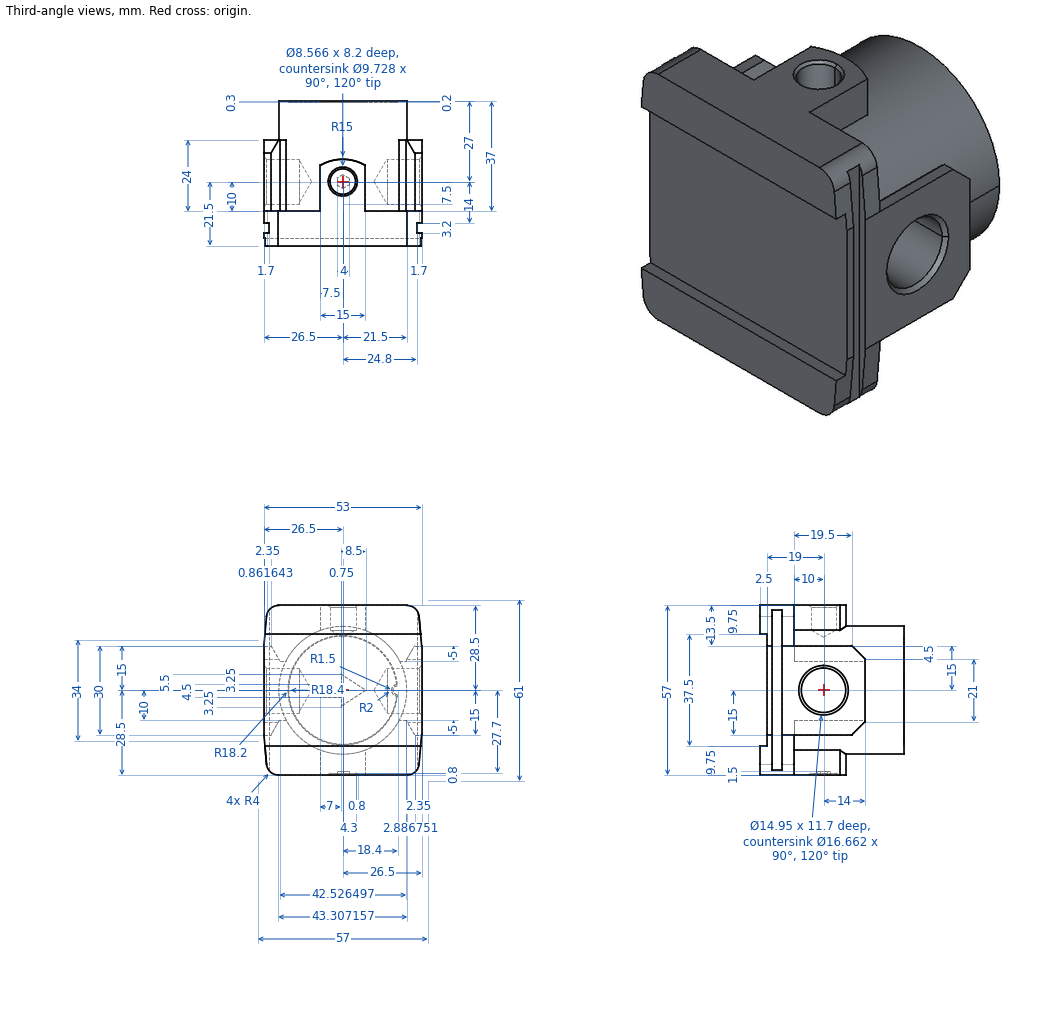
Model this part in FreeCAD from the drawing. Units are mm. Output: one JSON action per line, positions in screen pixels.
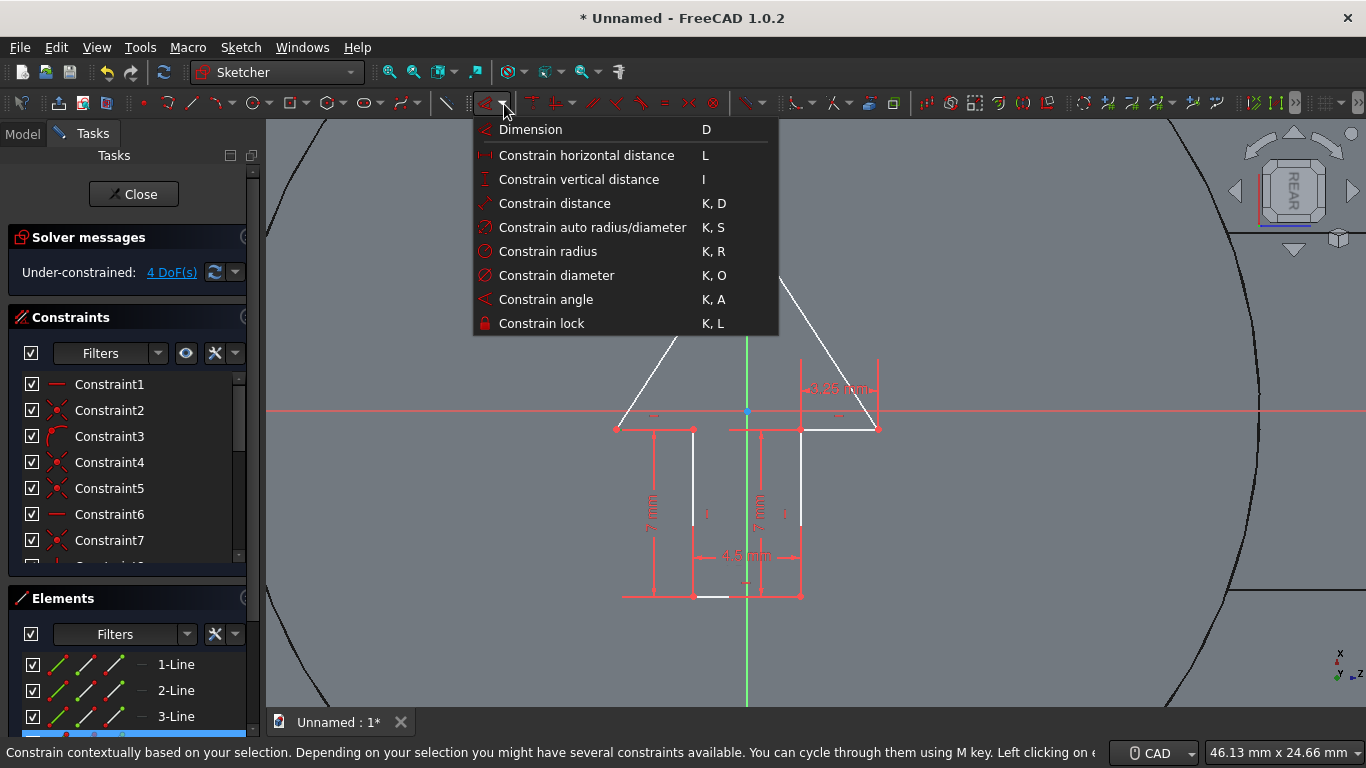
{"action": "left_click", "coordinate": [626, 155]}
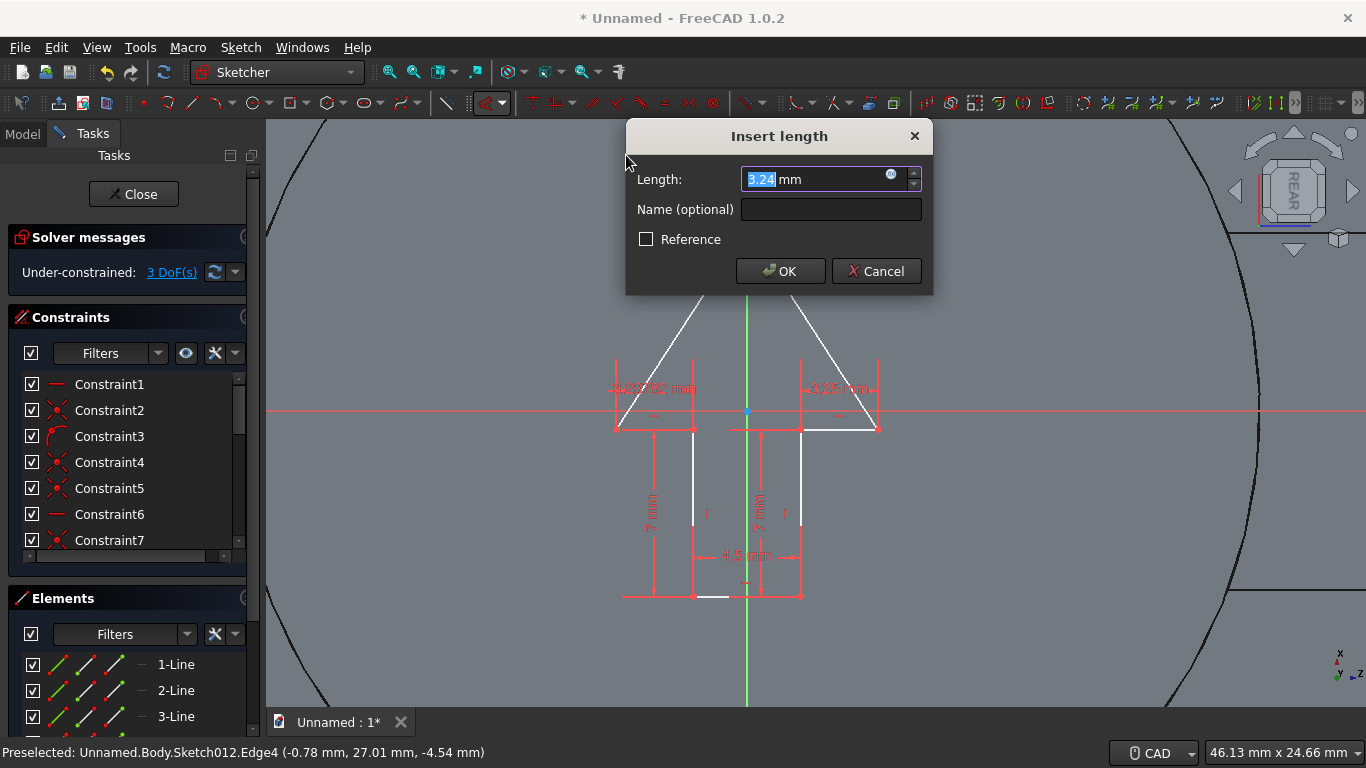
{"action": "type", "text": "3.25"}
{"action": "key", "text": "Return"}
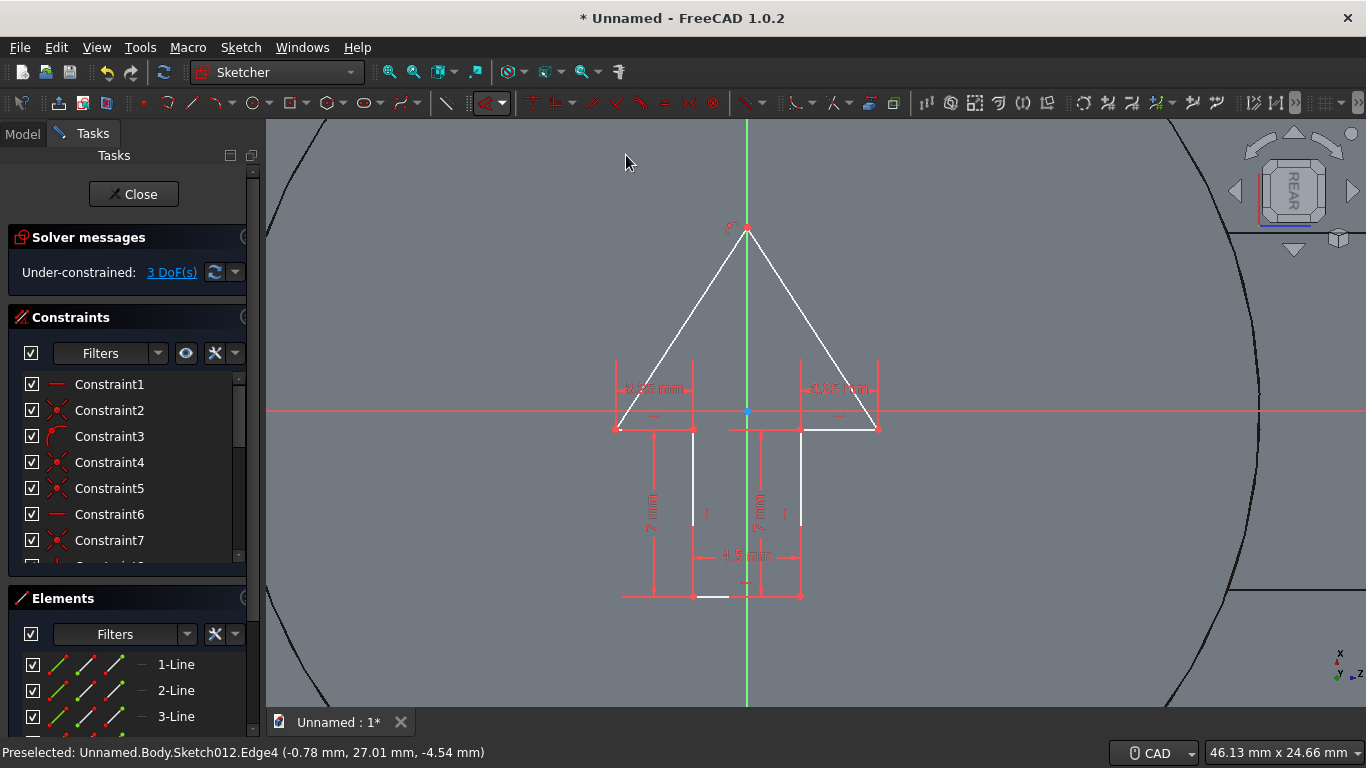
{"action": "left_click", "coordinate": [878, 430]}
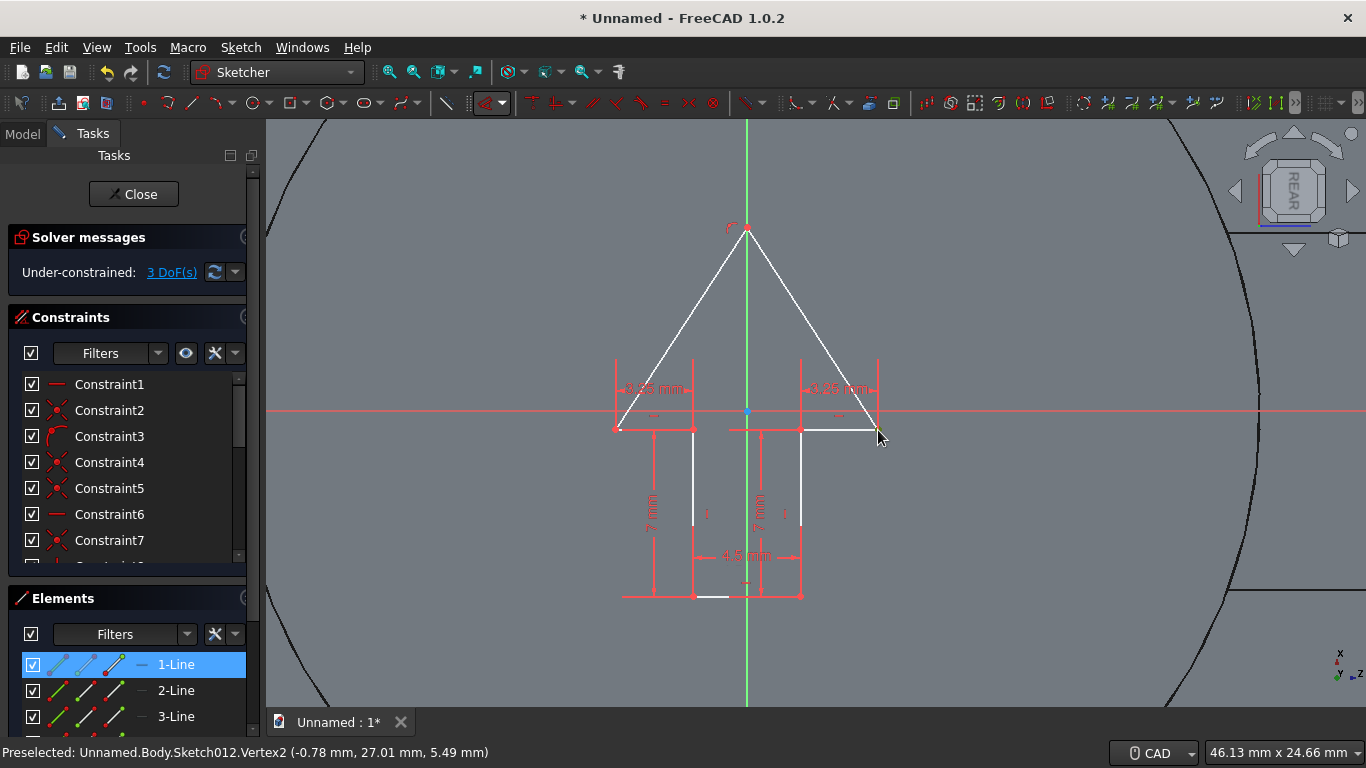
{"action": "key", "text": "l"}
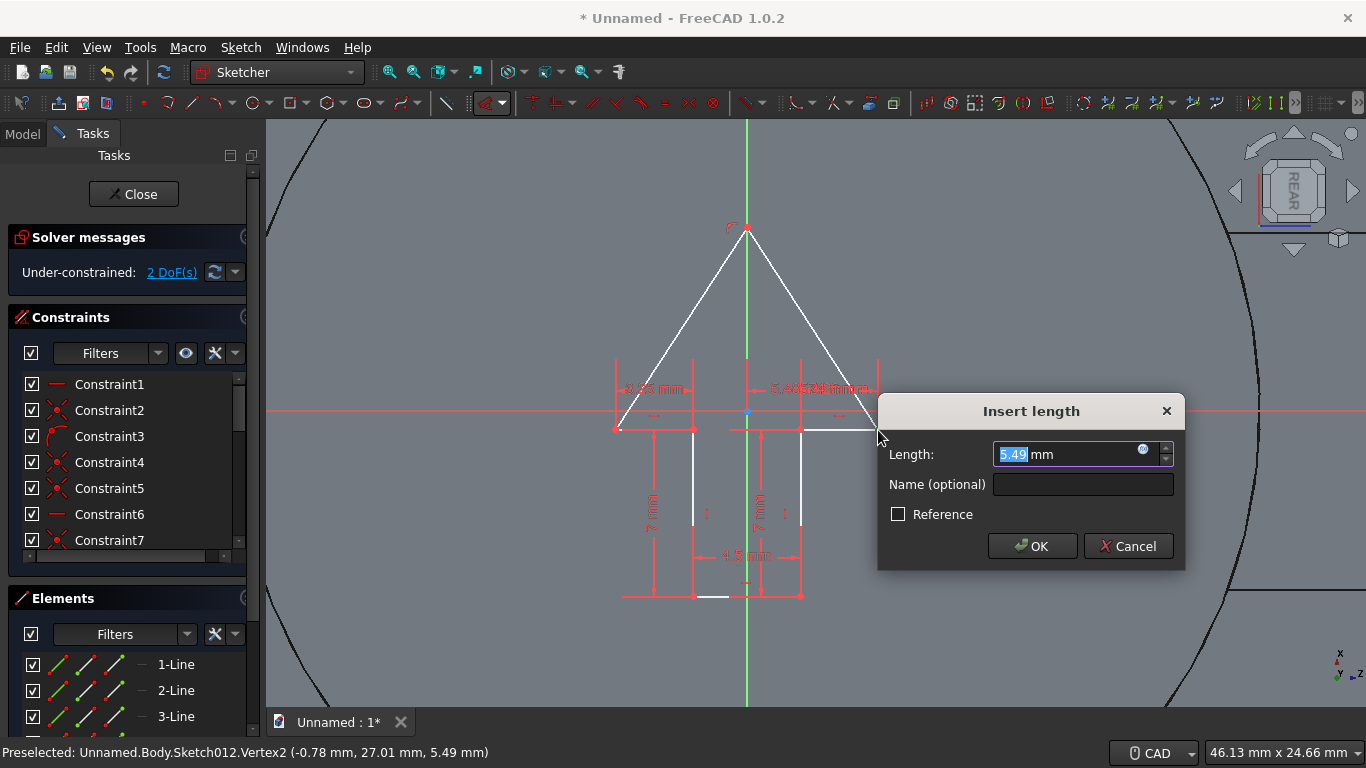
{"action": "type", "text": "5.5"}
{"action": "key", "text": "Return"}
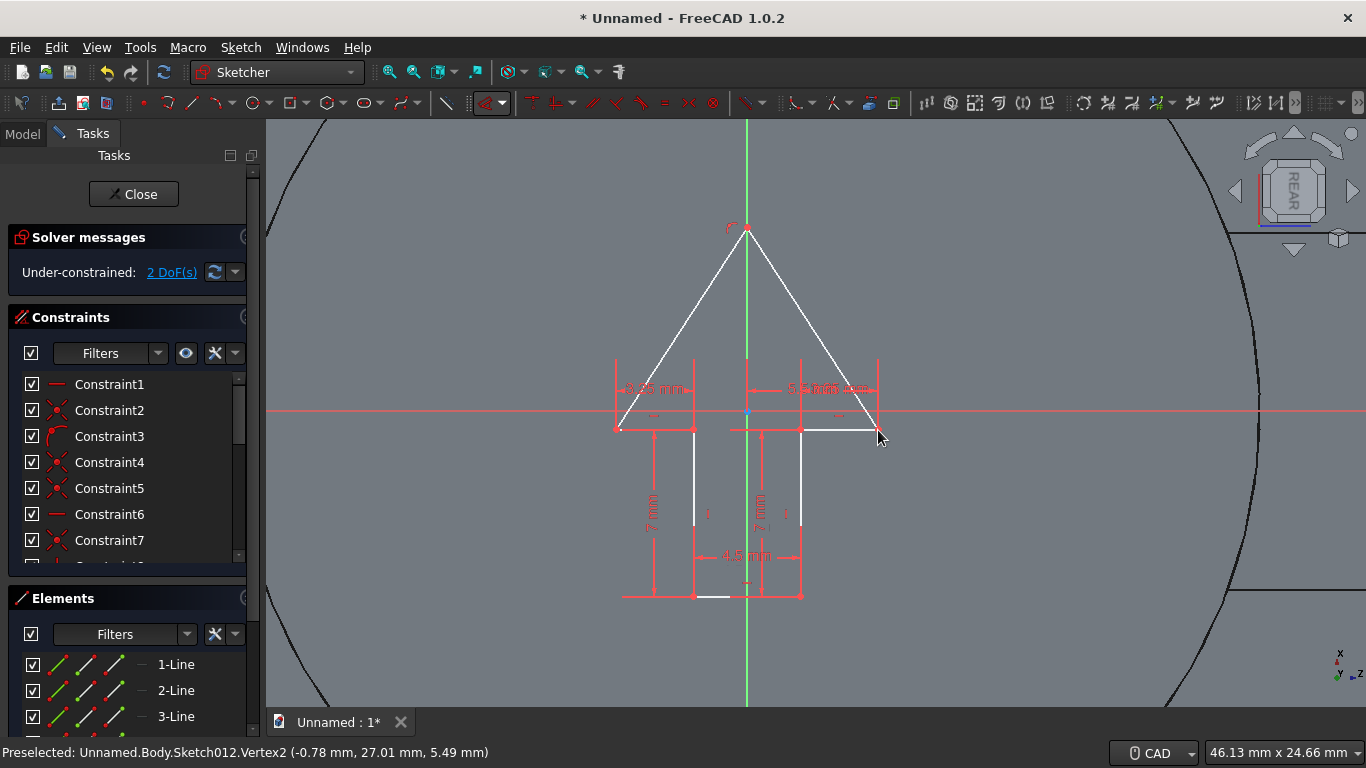
{"action": "left_click", "coordinate": [839, 369]}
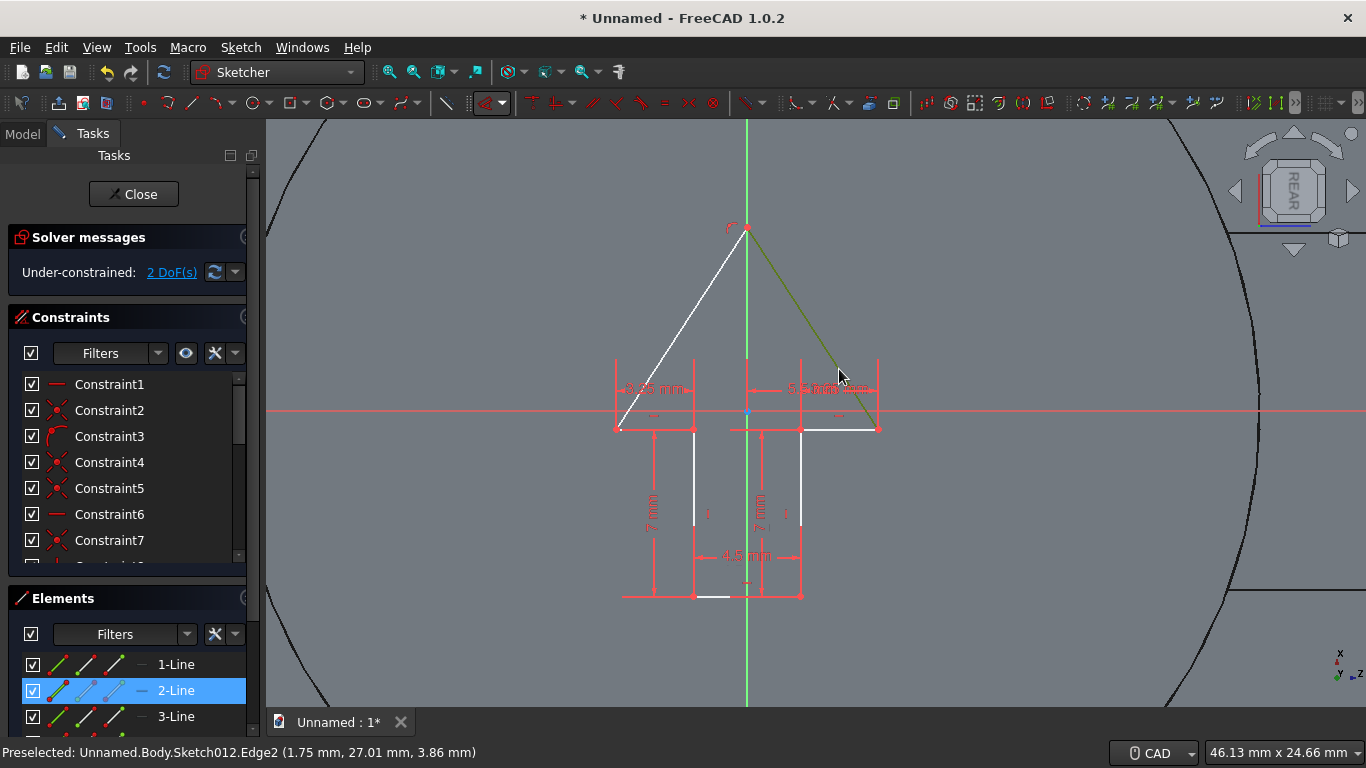
{"action": "key", "text": "i"}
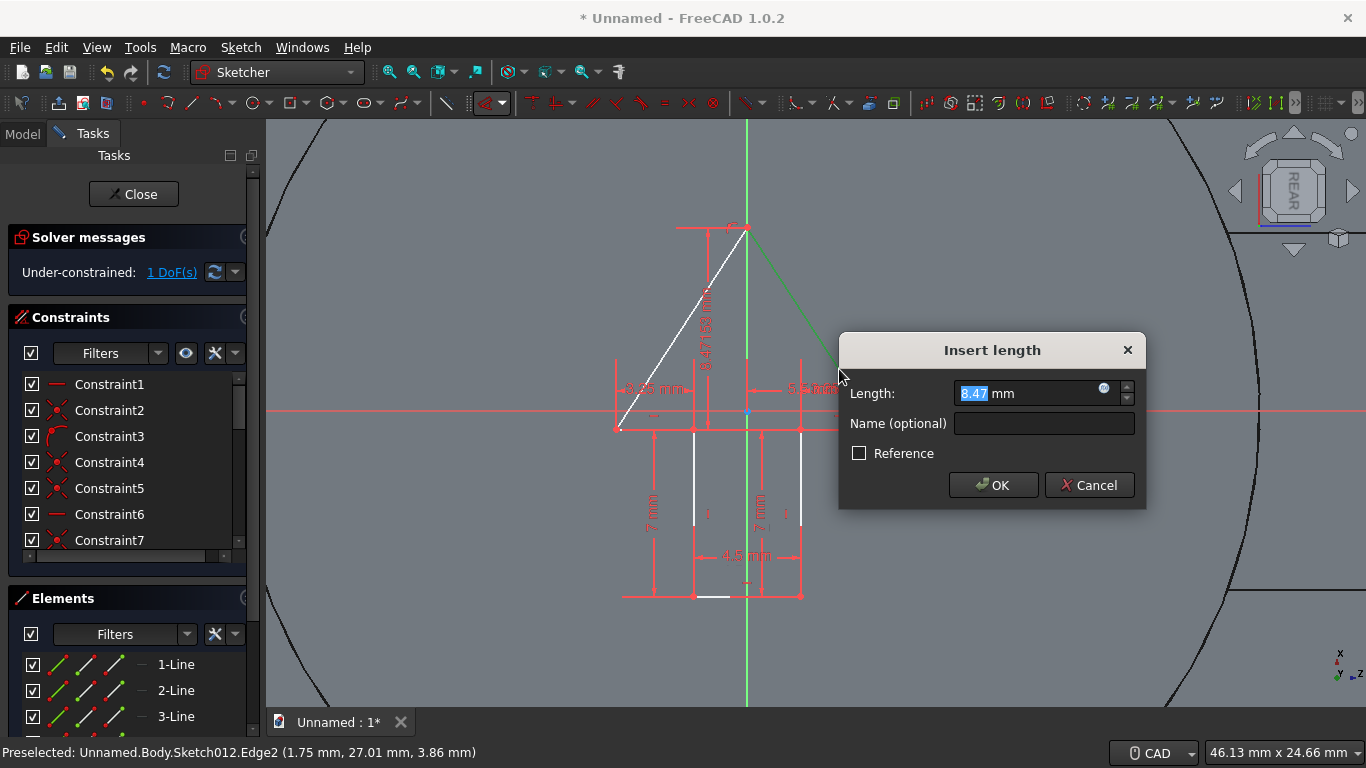
{"action": "type", "text": "8.5"}
{"action": "key", "text": "Return"}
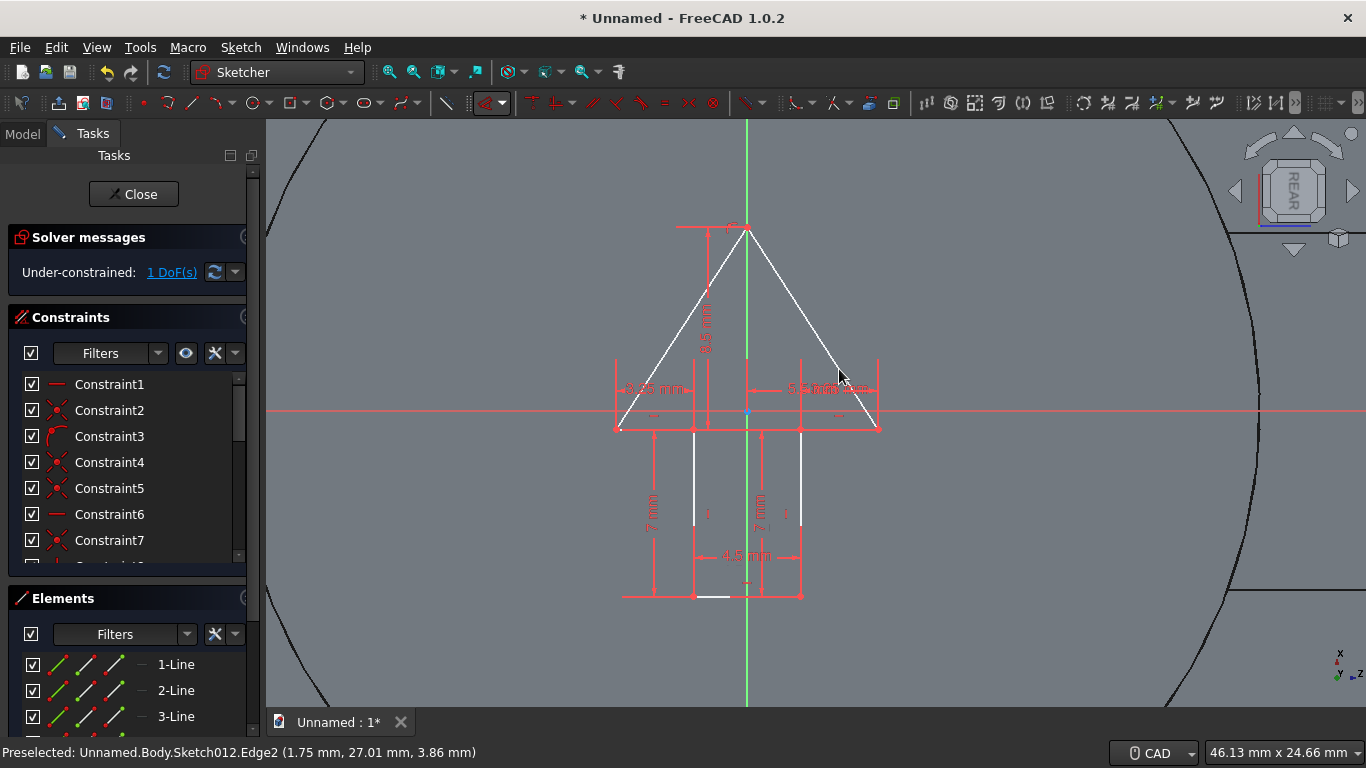
{"action": "scroll", "coordinate": [801, 430], "scroll_direction": "up", "scroll_amount": 4}